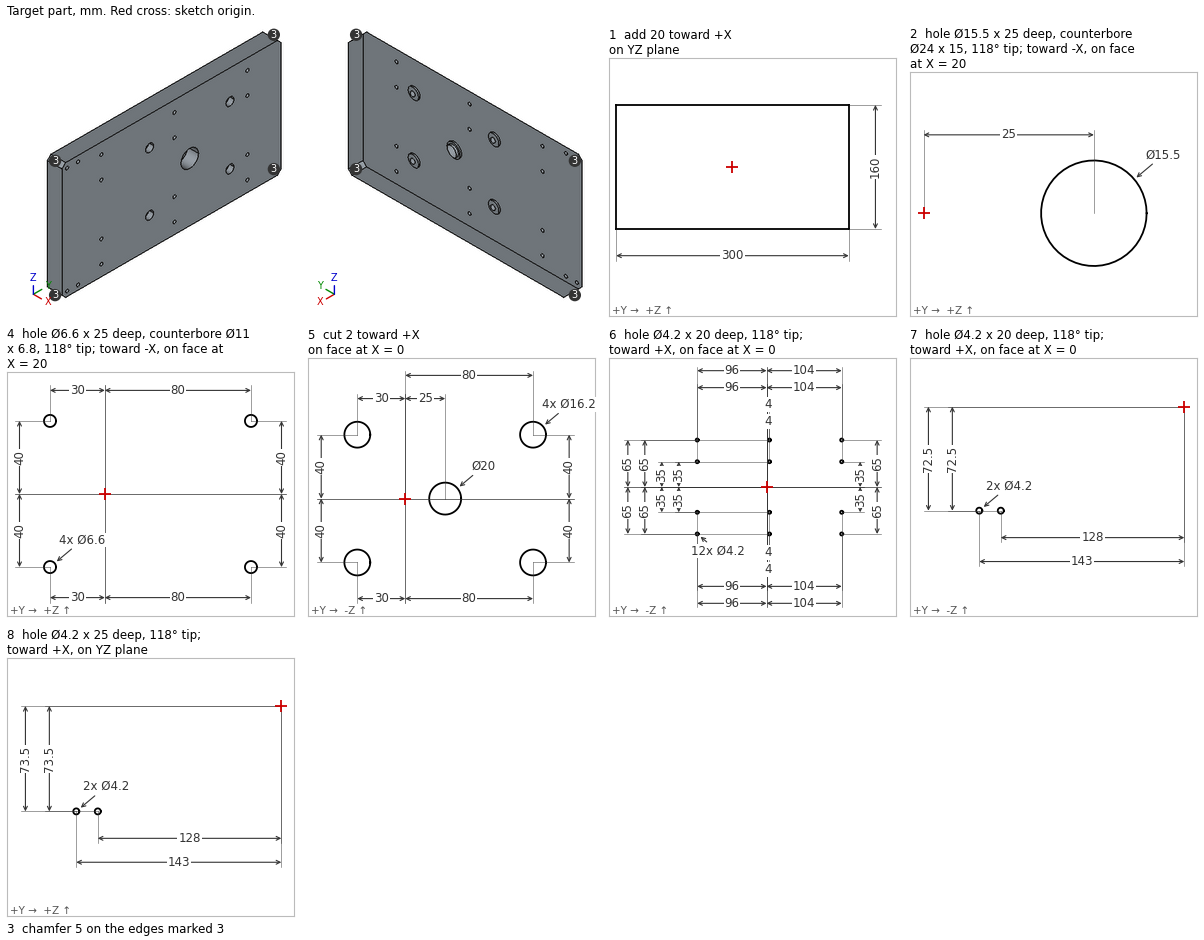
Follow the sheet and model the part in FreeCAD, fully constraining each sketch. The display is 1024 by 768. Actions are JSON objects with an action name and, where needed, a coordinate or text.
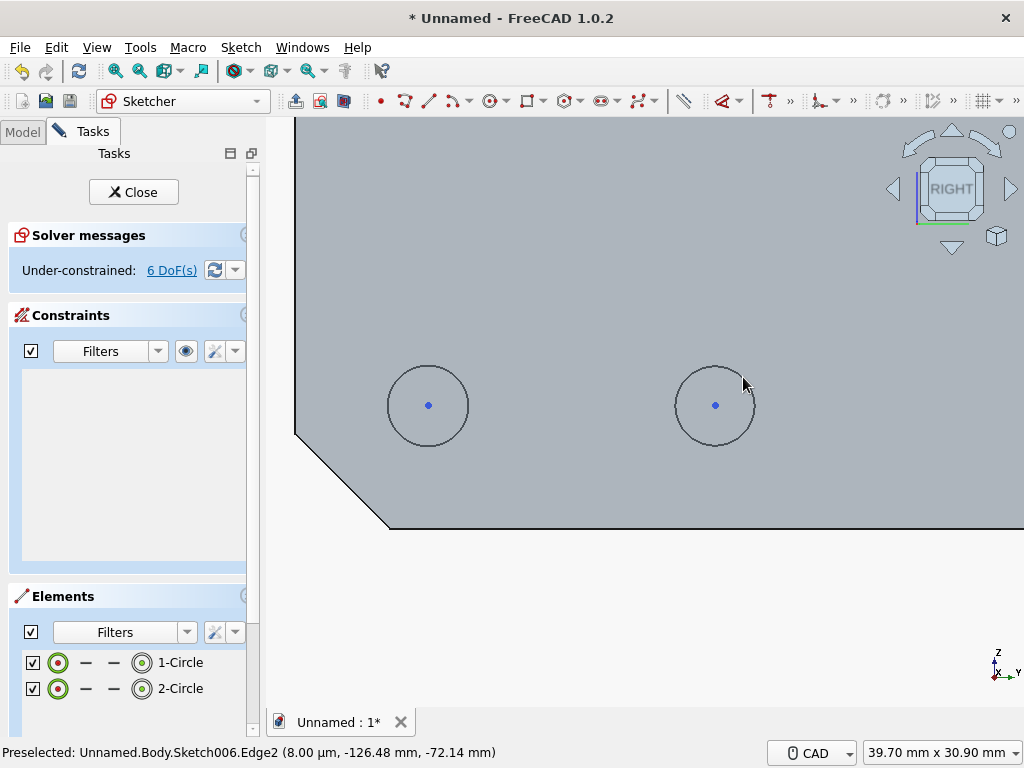
{"action": "left_click", "coordinate": [456, 377]}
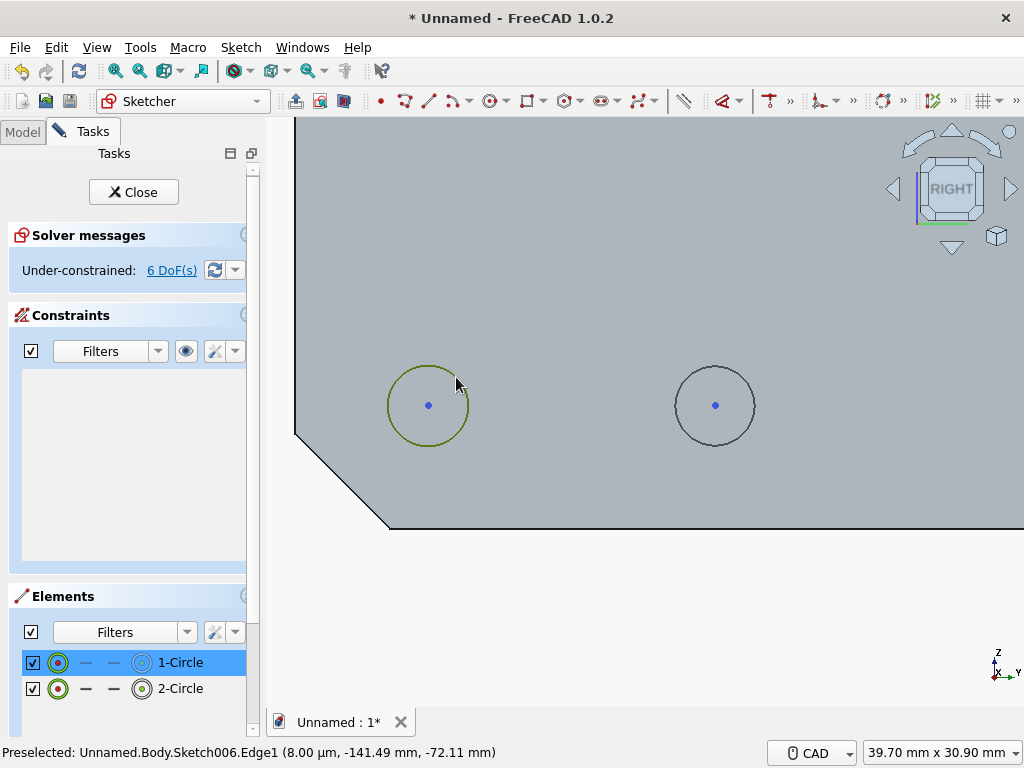
{"action": "left_click", "coordinate": [743, 378]}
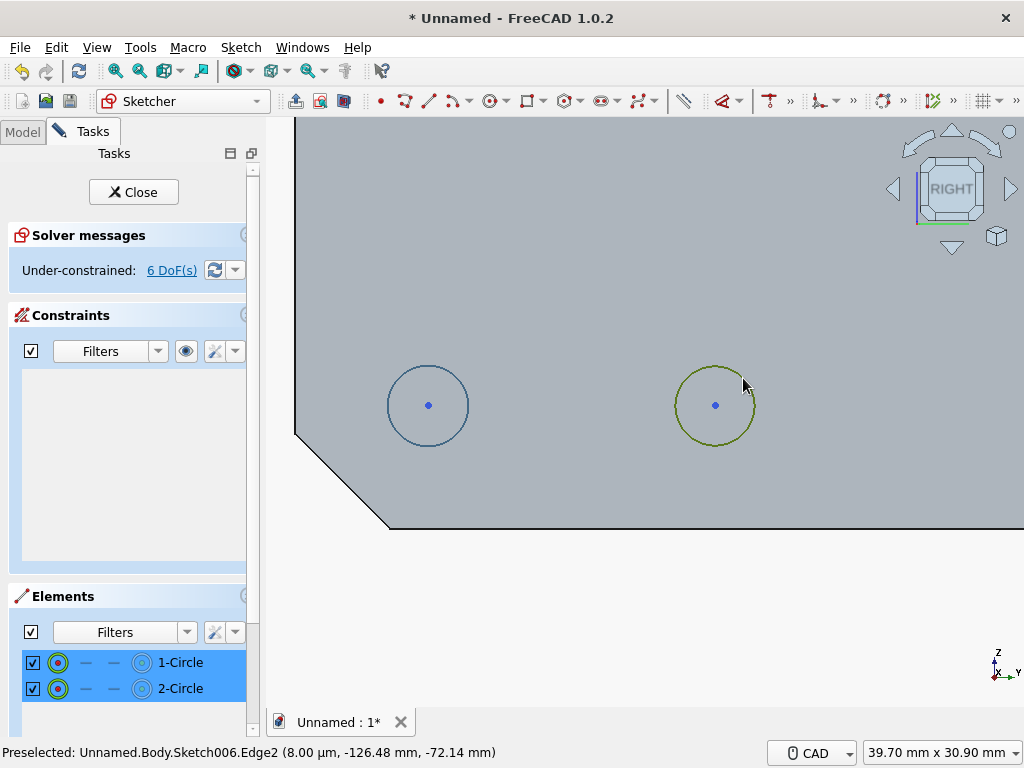
{"action": "key", "text": "e"}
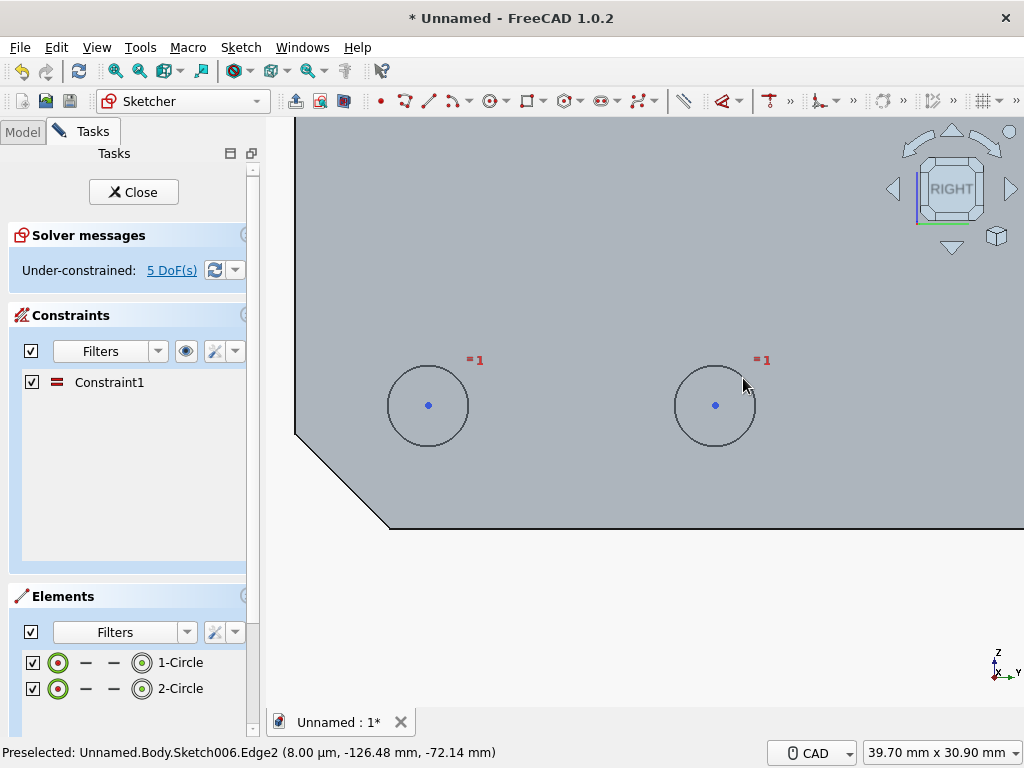
{"action": "left_click", "coordinate": [722, 102]}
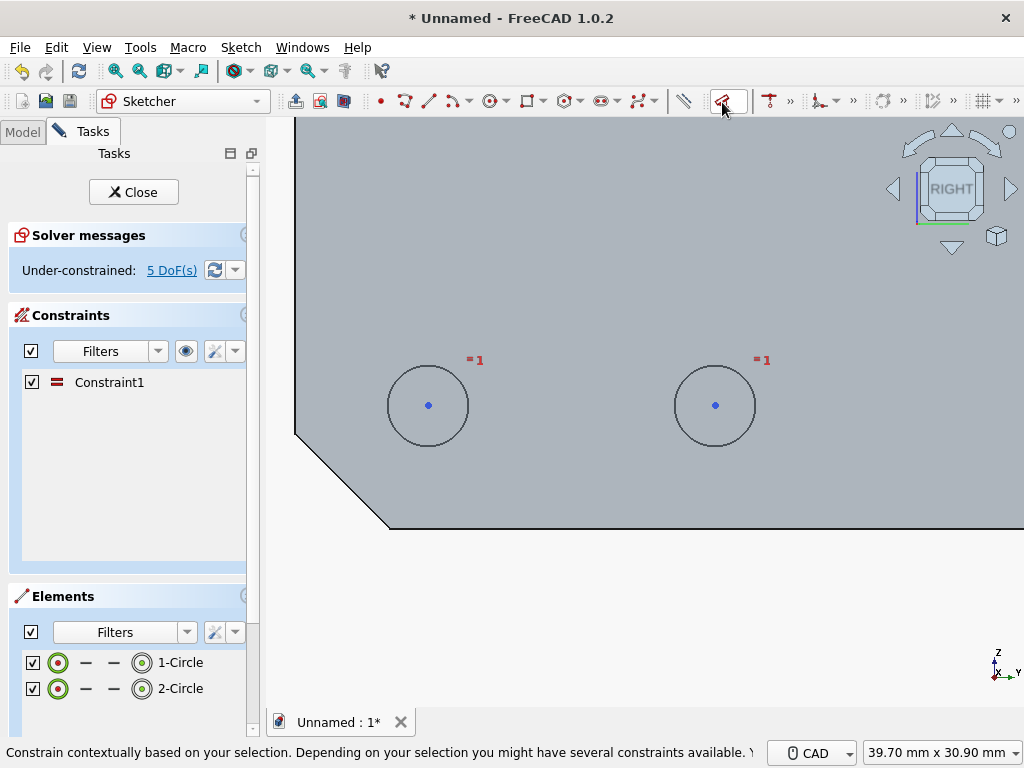
{"action": "left_click", "coordinate": [456, 377]}
{"action": "left_click", "coordinate": [478, 354]}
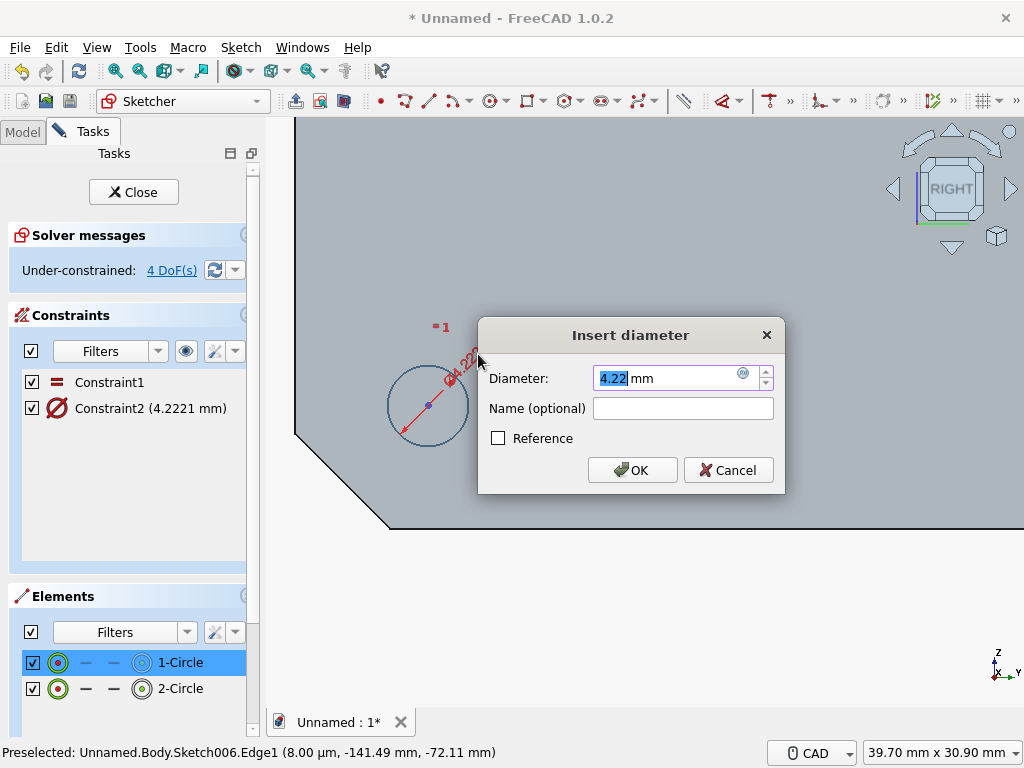
{"action": "type", "text": "4.2"}
{"action": "key", "text": "Return"}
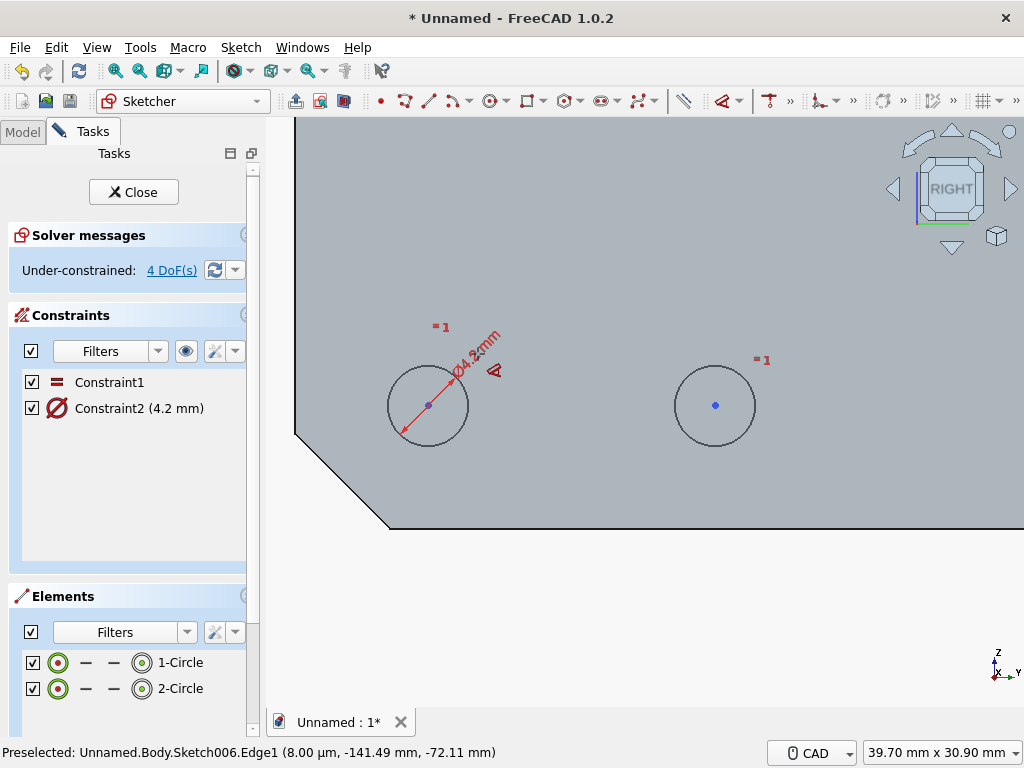
{"action": "left_click", "coordinate": [428, 406]}
{"action": "left_click", "coordinate": [644, 440]}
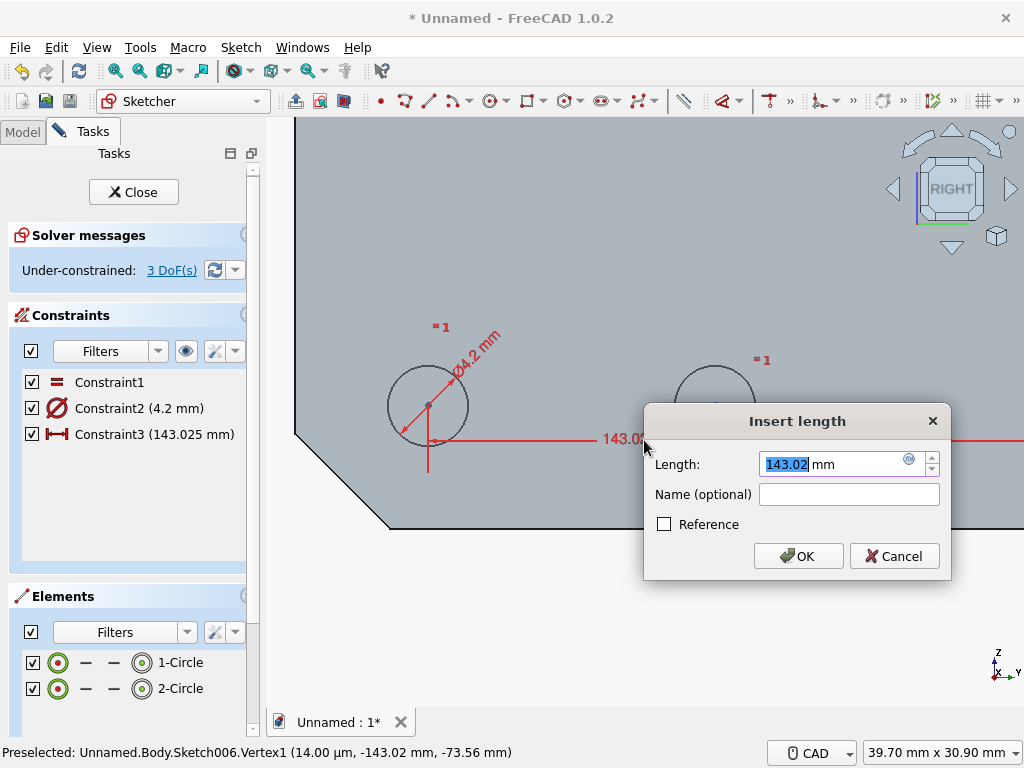
{"action": "type", "text": "143"}
{"action": "key", "text": "Return"}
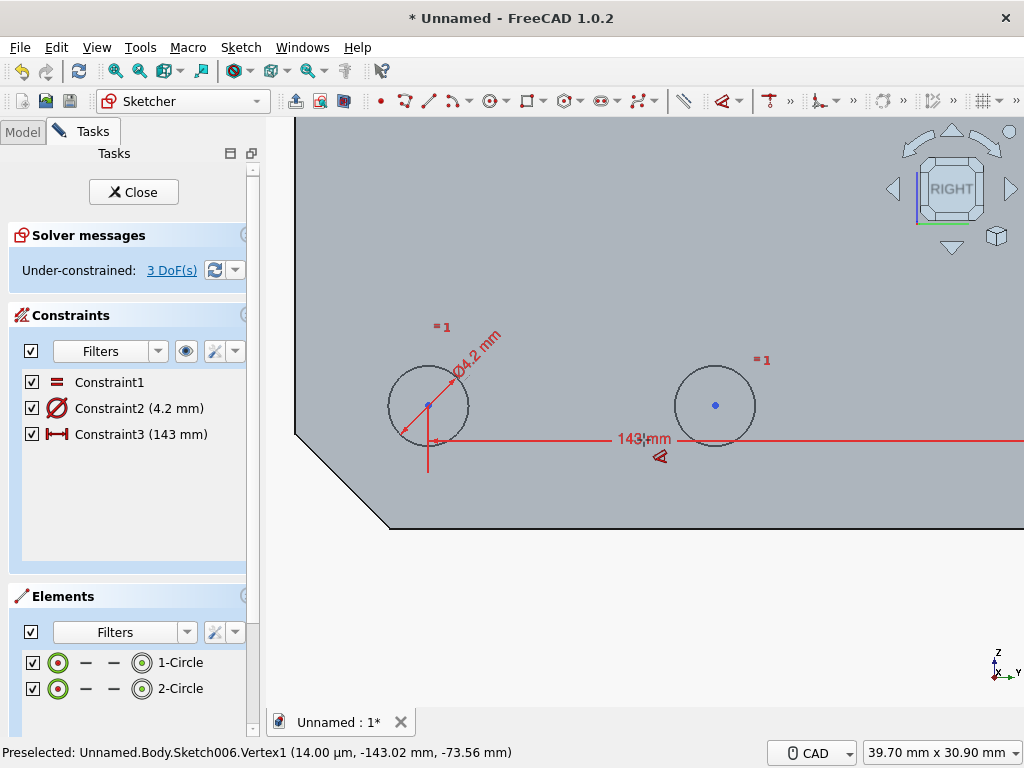
{"action": "left_click", "coordinate": [715, 406]}
{"action": "left_click", "coordinate": [787, 440]}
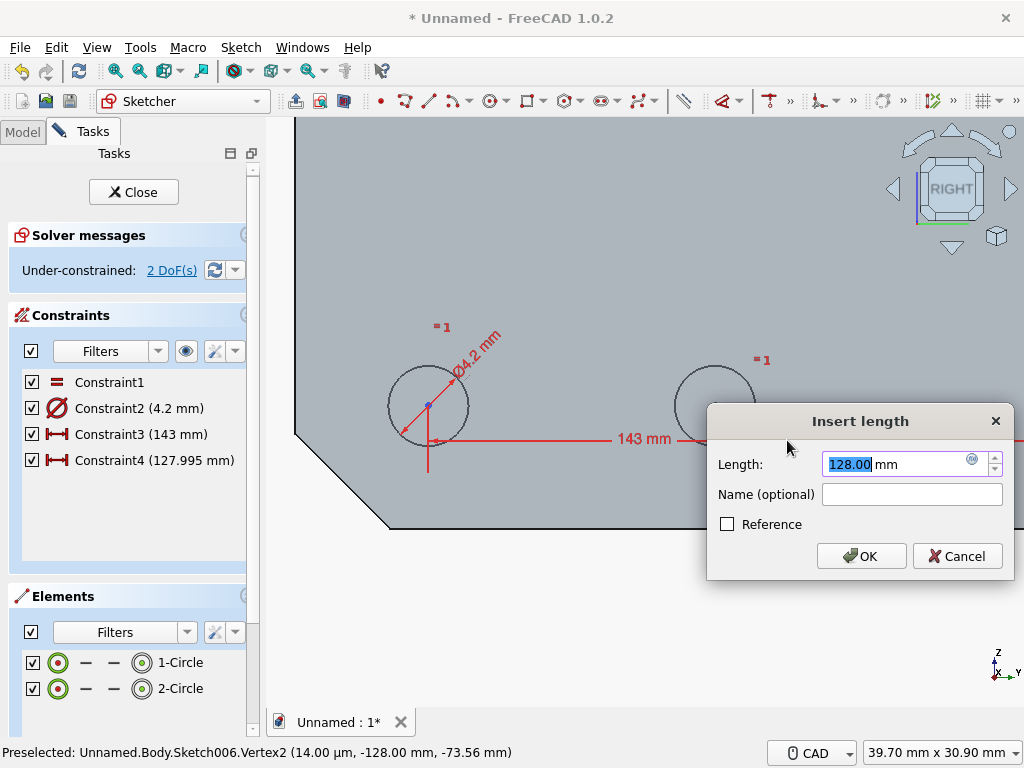
{"action": "type", "text": "128"}
{"action": "key", "text": "Return"}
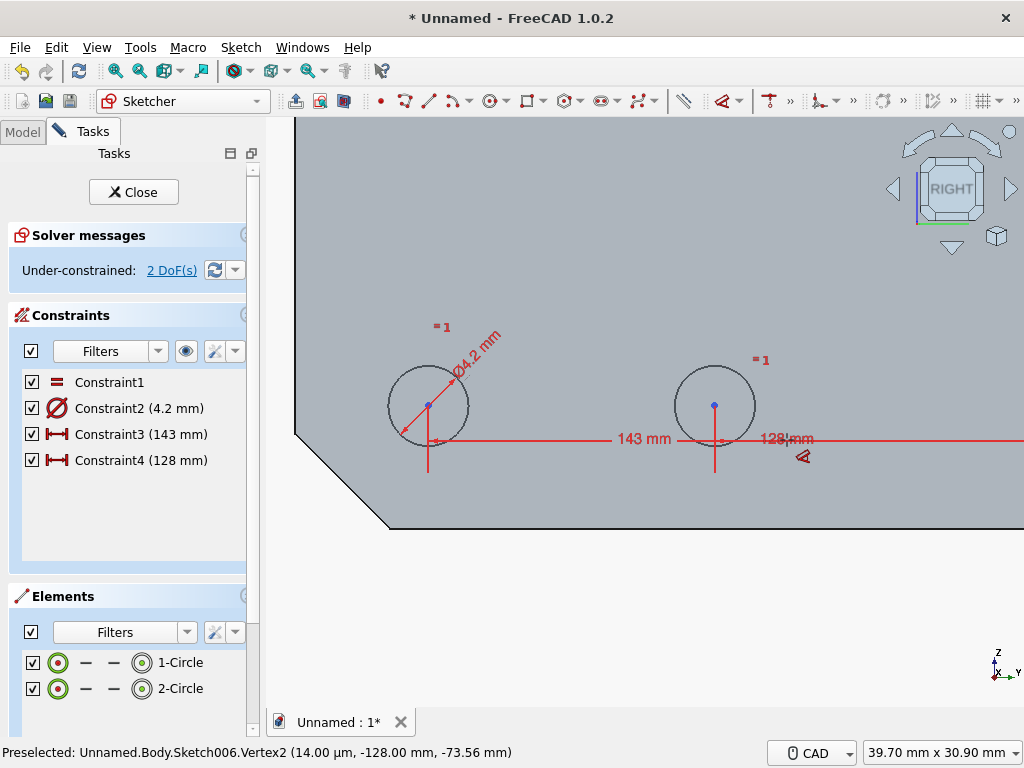
{"action": "left_click", "coordinate": [428, 406]}
{"action": "left_click", "coordinate": [394, 276]}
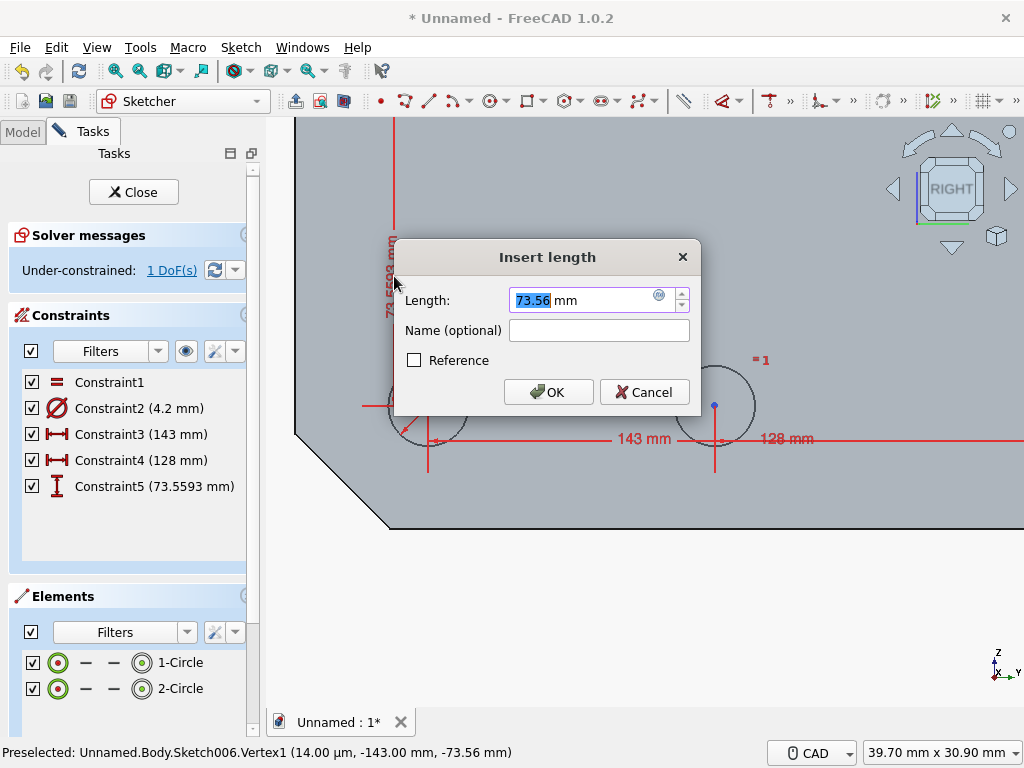
{"action": "type", "text": "73.5"}
{"action": "key", "text": "Return"}